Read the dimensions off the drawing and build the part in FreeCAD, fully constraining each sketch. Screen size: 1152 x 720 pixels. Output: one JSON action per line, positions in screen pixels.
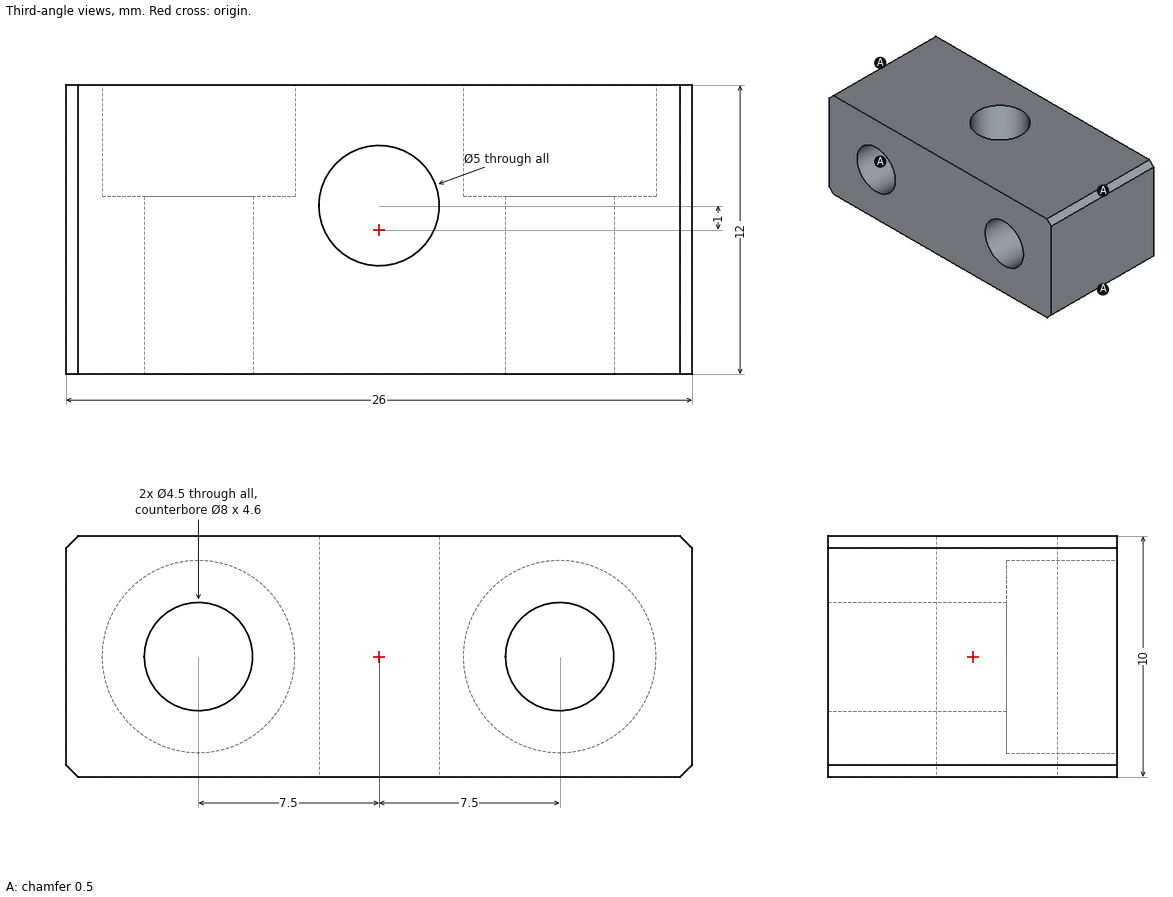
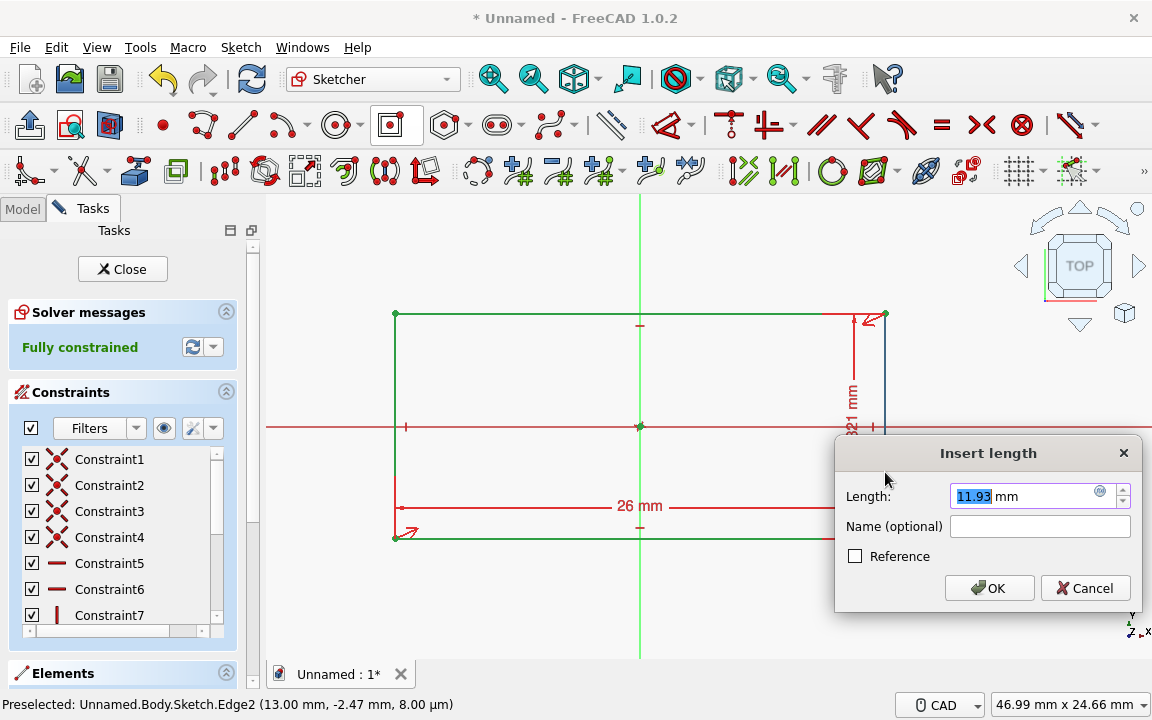
{"action": "type", "text": "12"}
{"action": "key", "text": "Return"}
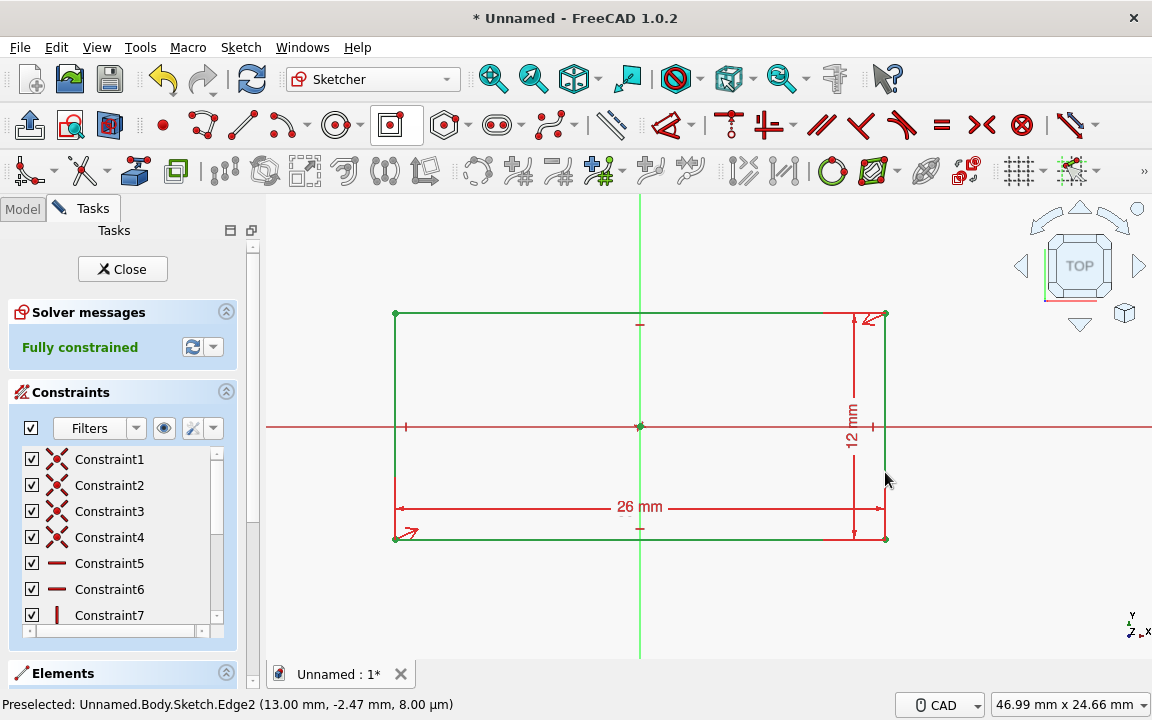
{"action": "left_click", "coordinate": [123, 269]}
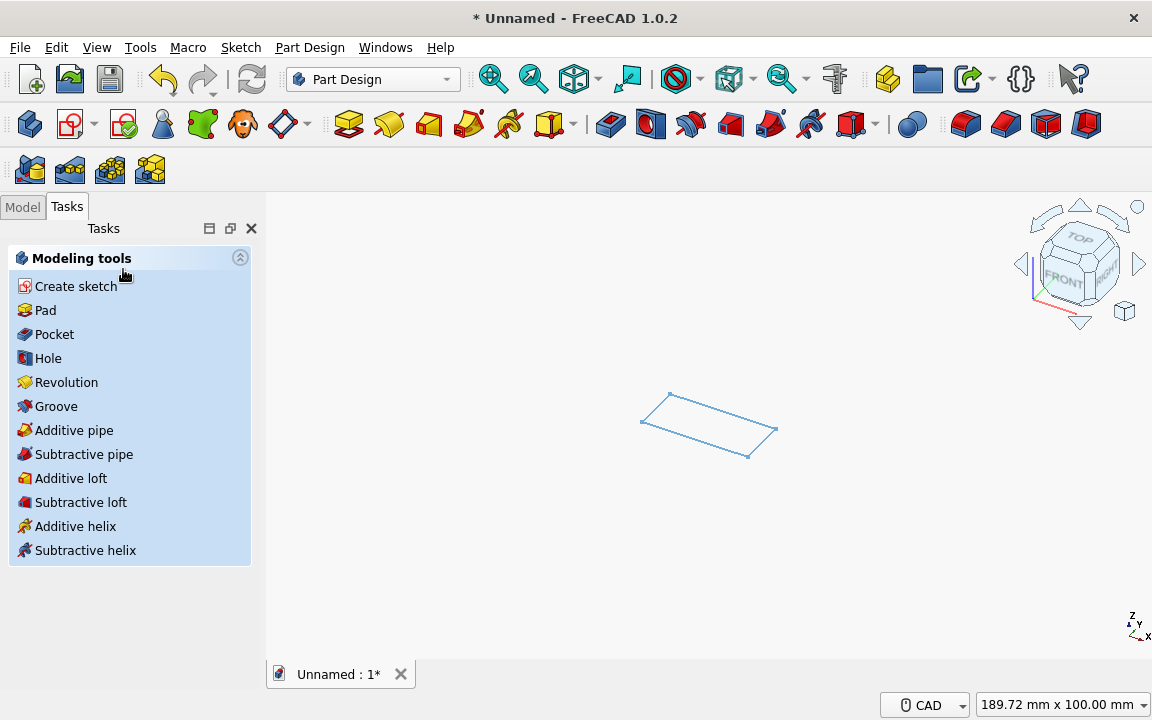
{"action": "left_click", "coordinate": [350, 124]}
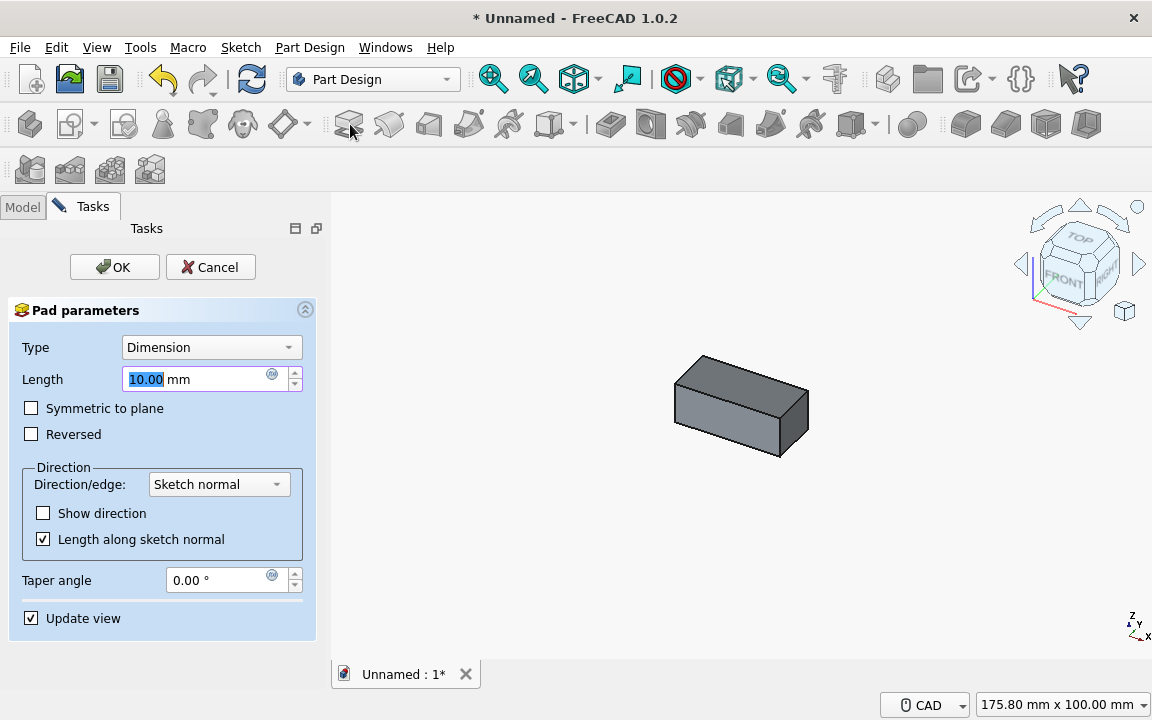
{"action": "type", "text": "10"}
{"action": "key", "text": "Tab"}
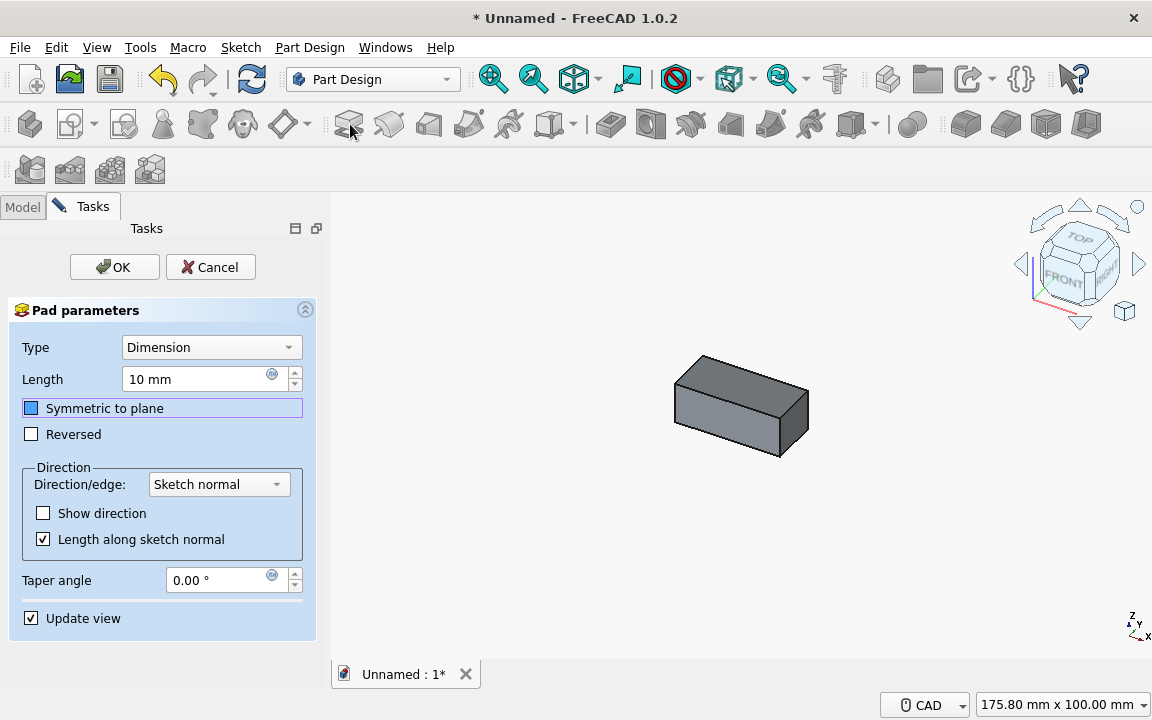
{"action": "left_click", "coordinate": [30, 408]}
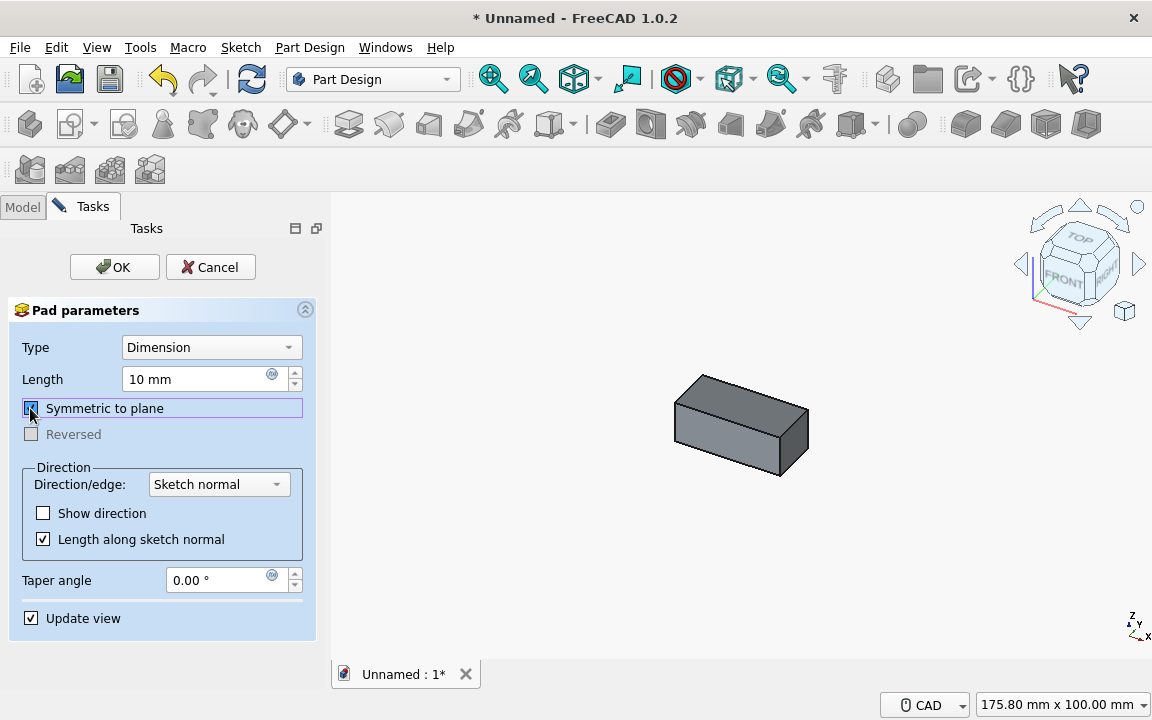
{"action": "left_click", "coordinate": [115, 267]}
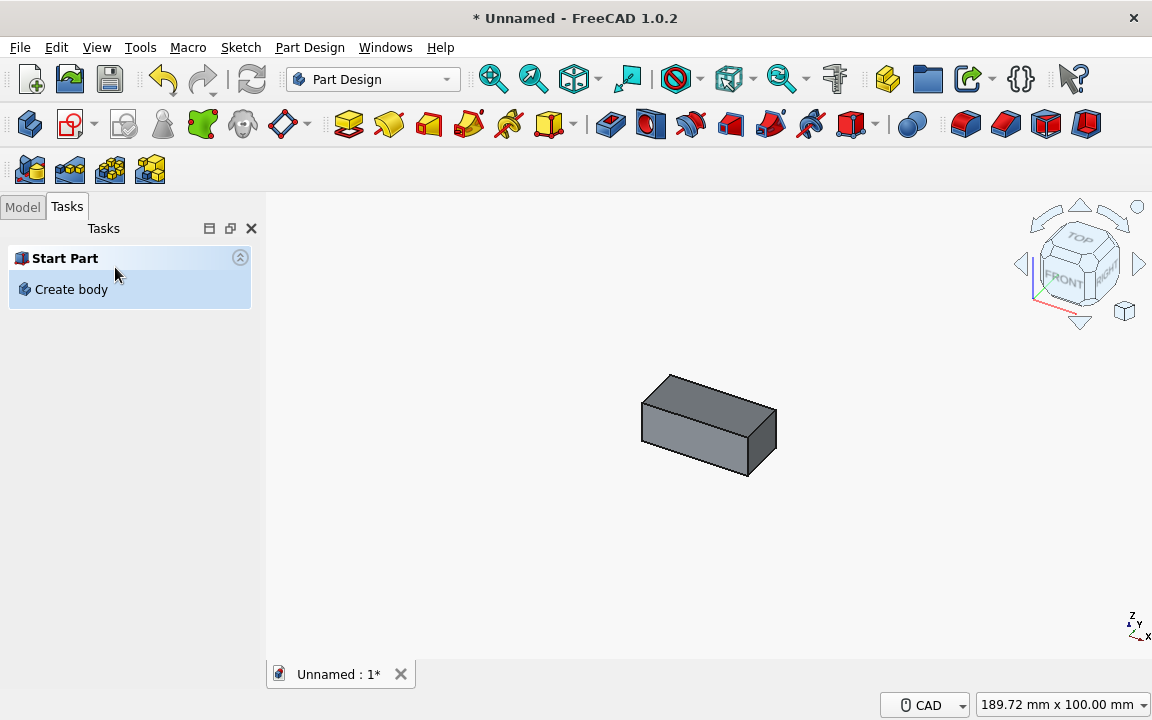
{"action": "key", "text": "v f"}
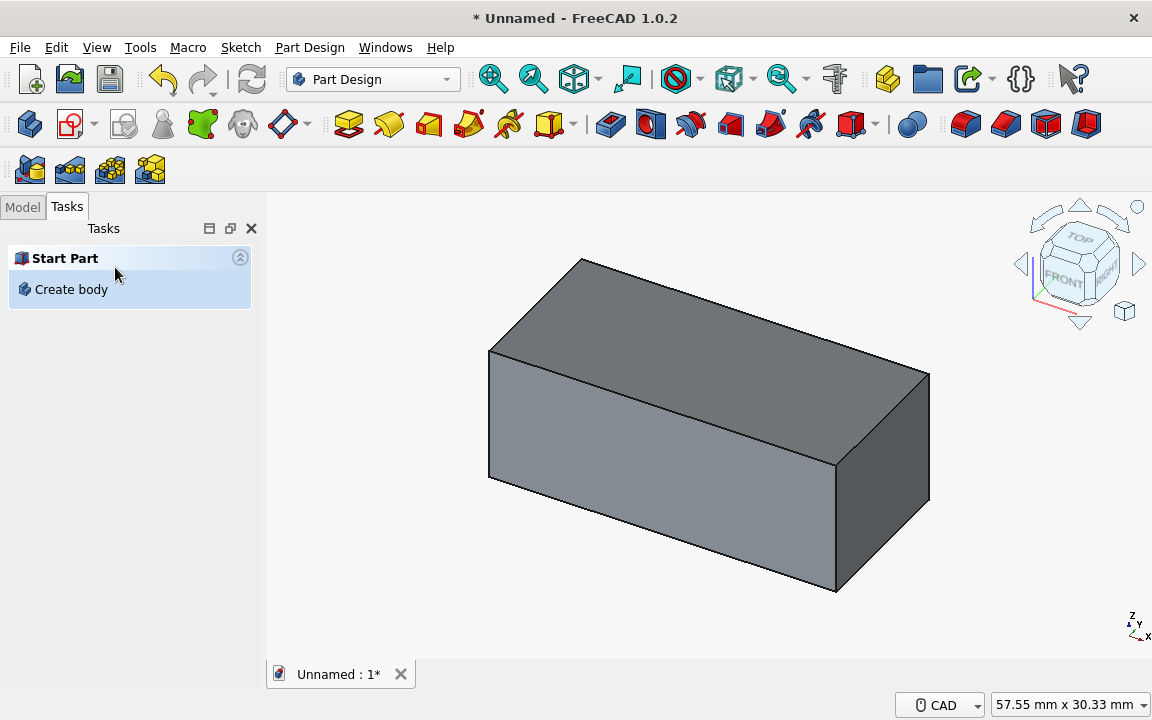
{"action": "key", "text": "4"}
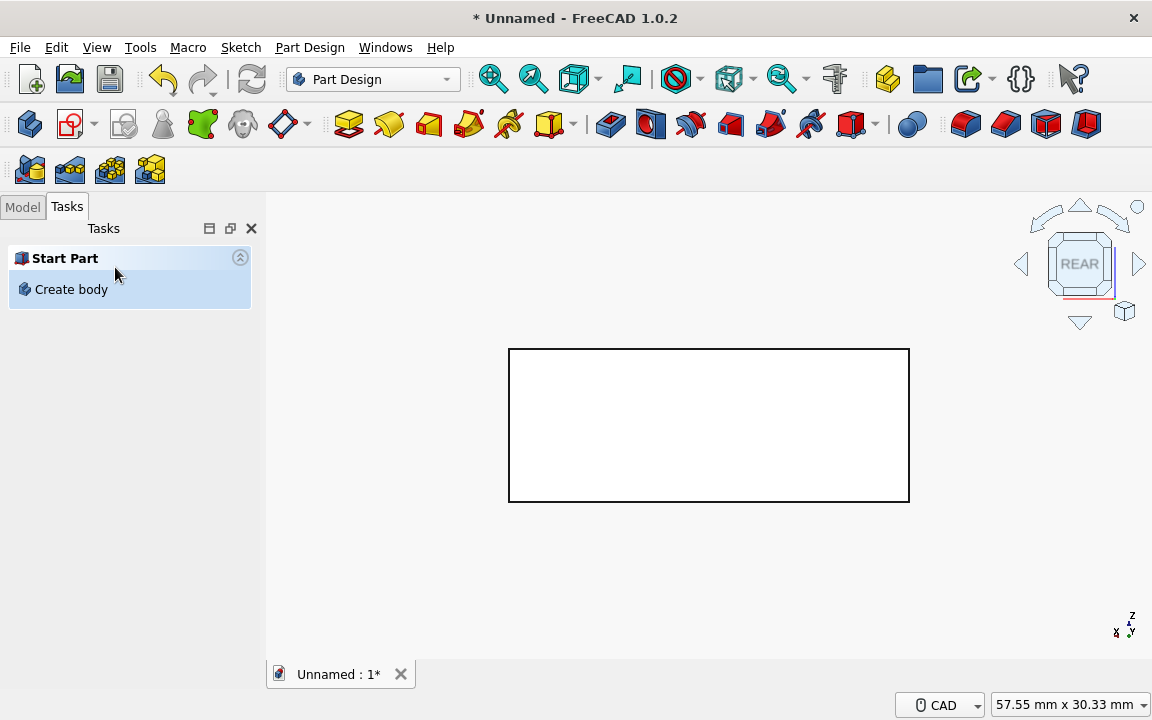
{"action": "left_click", "coordinate": [595, 425]}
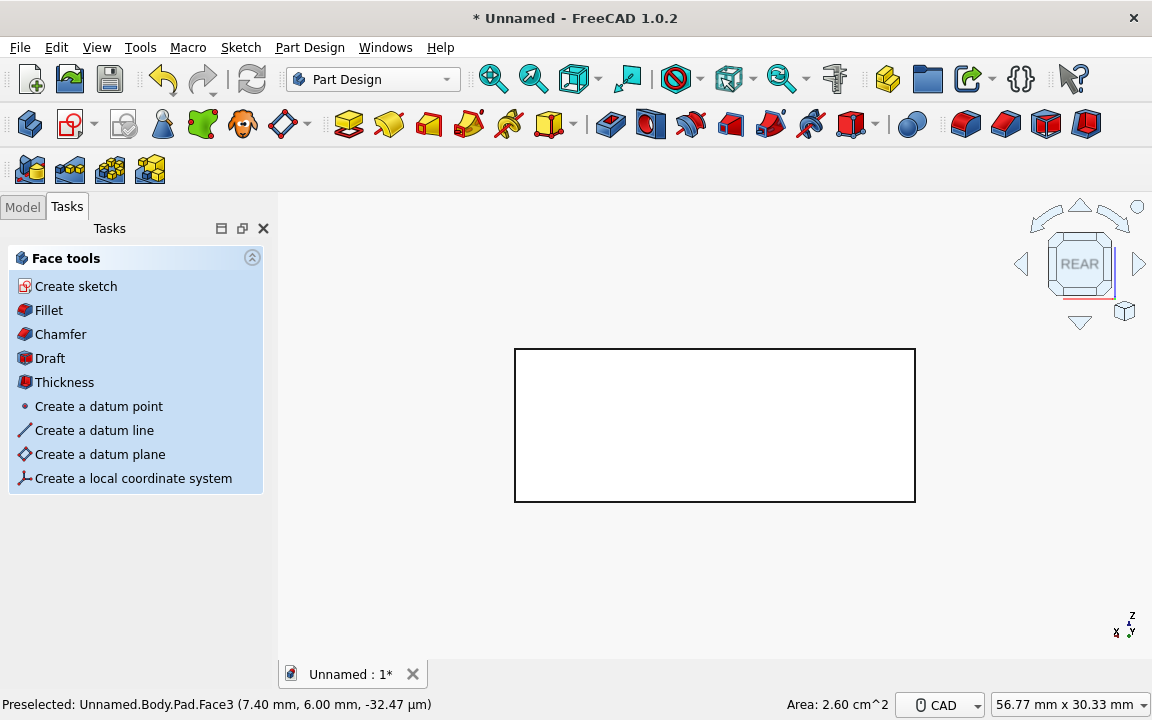
{"action": "left_click", "coordinate": [70, 124]}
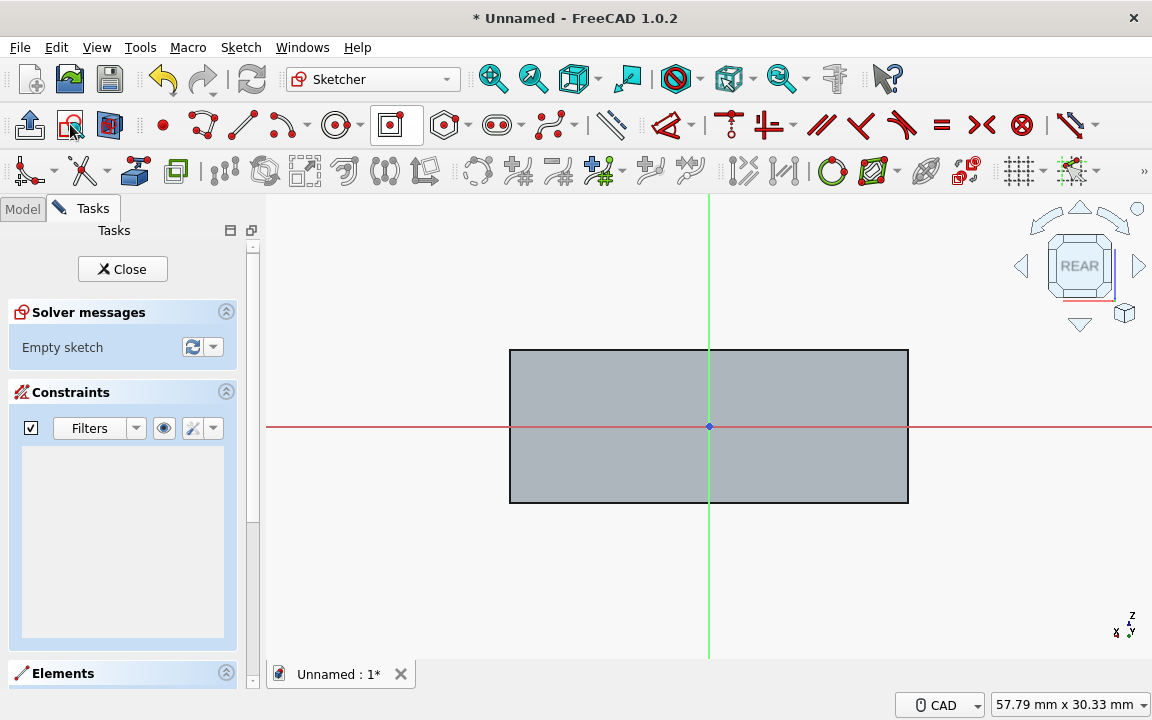
{"action": "scroll", "coordinate": [848, 427], "scroll_direction": "up", "scroll_amount": 2}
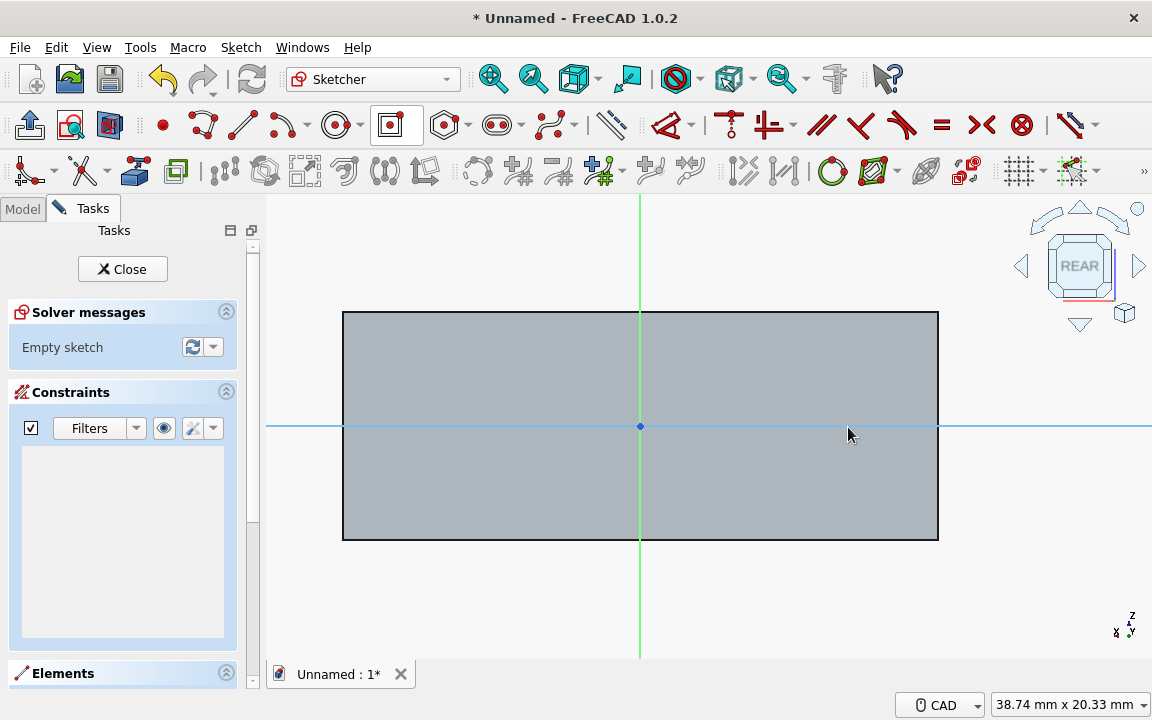
{"action": "key", "text": "g c"}